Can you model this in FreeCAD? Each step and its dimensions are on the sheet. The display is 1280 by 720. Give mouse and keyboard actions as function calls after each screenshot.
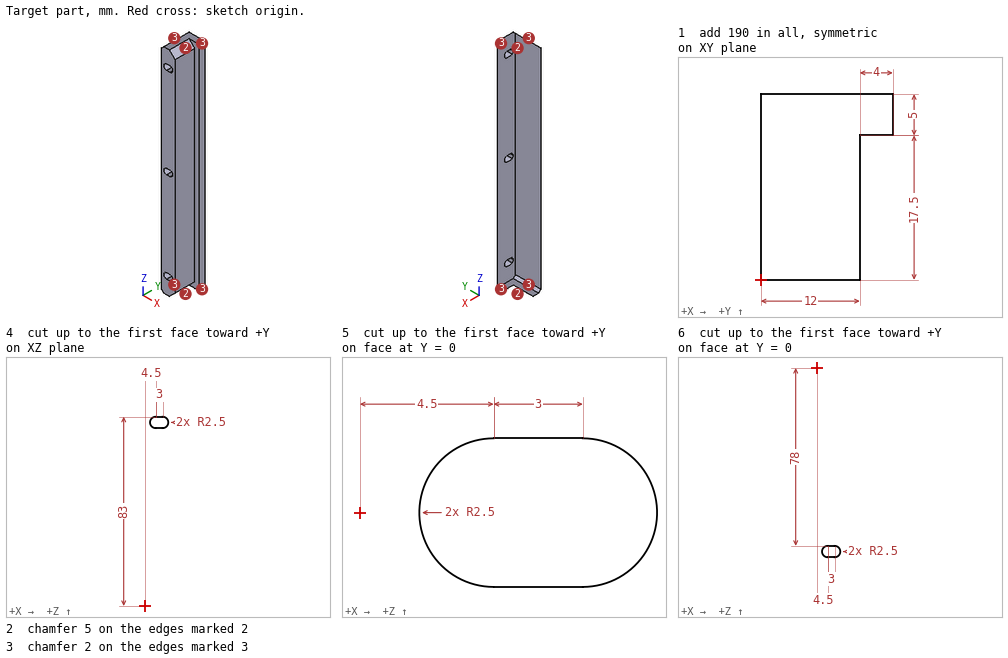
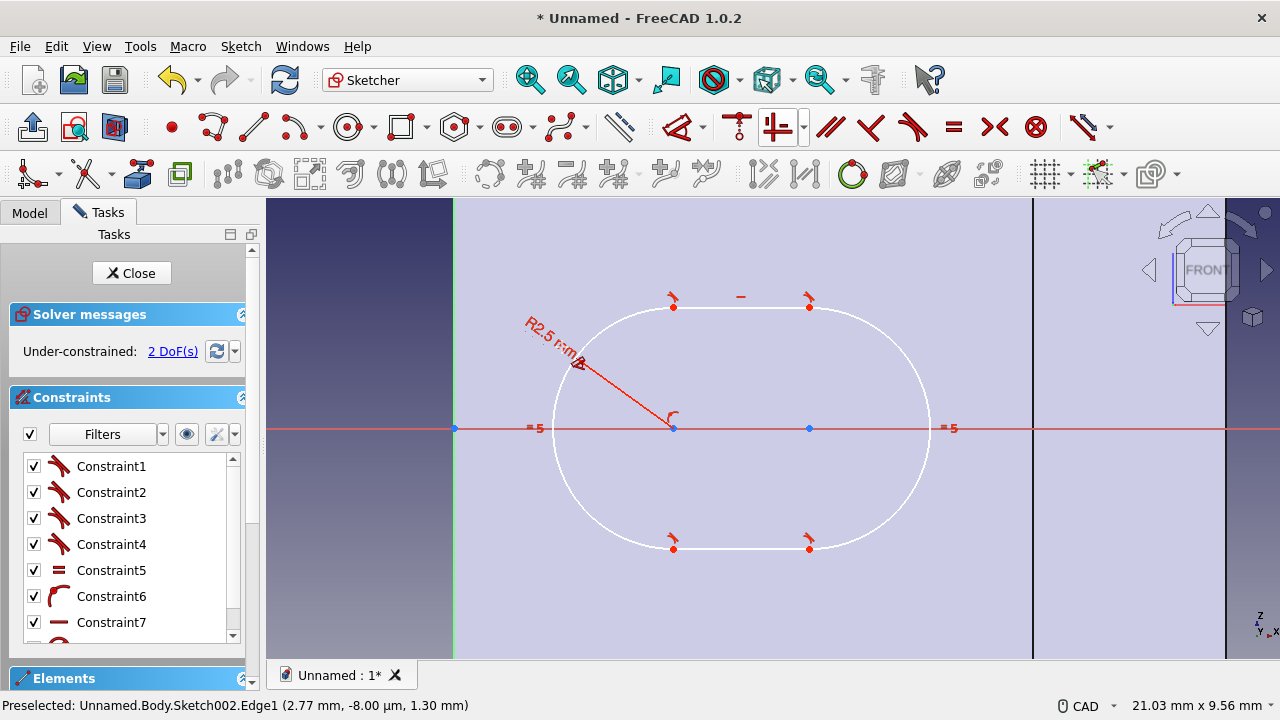
click(714, 308)
click(742, 274)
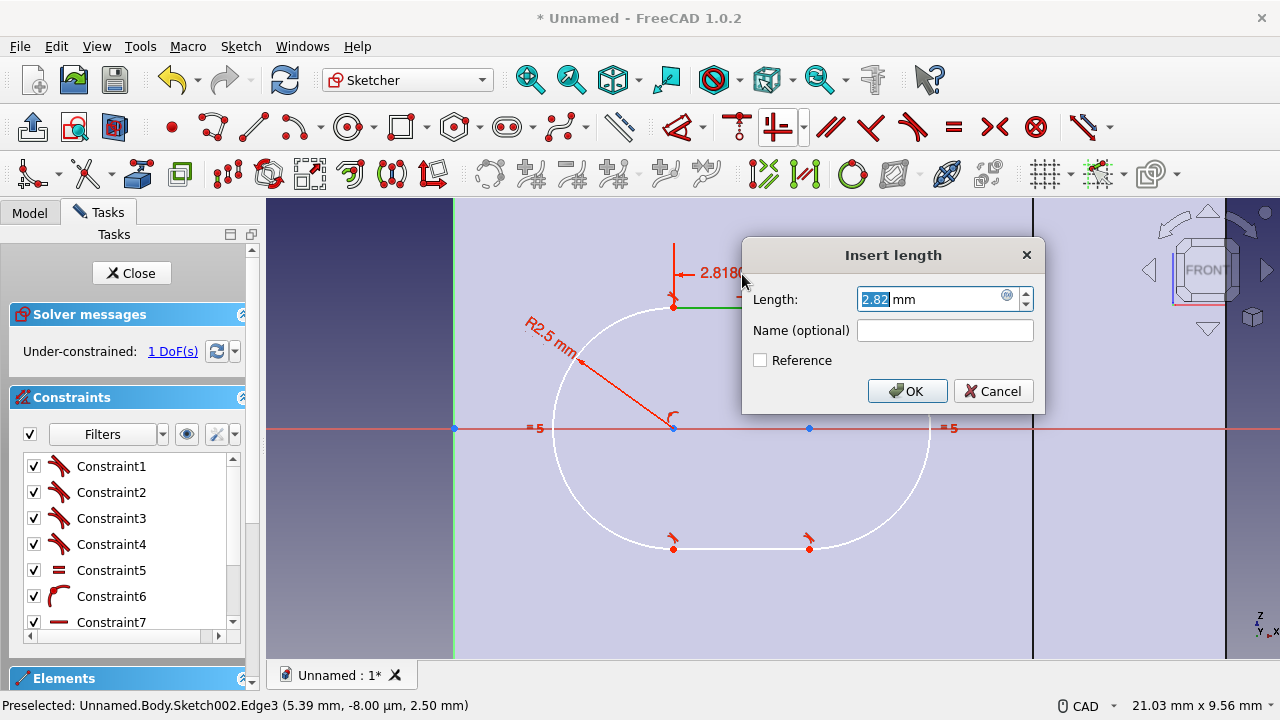
text(3)
key(Return)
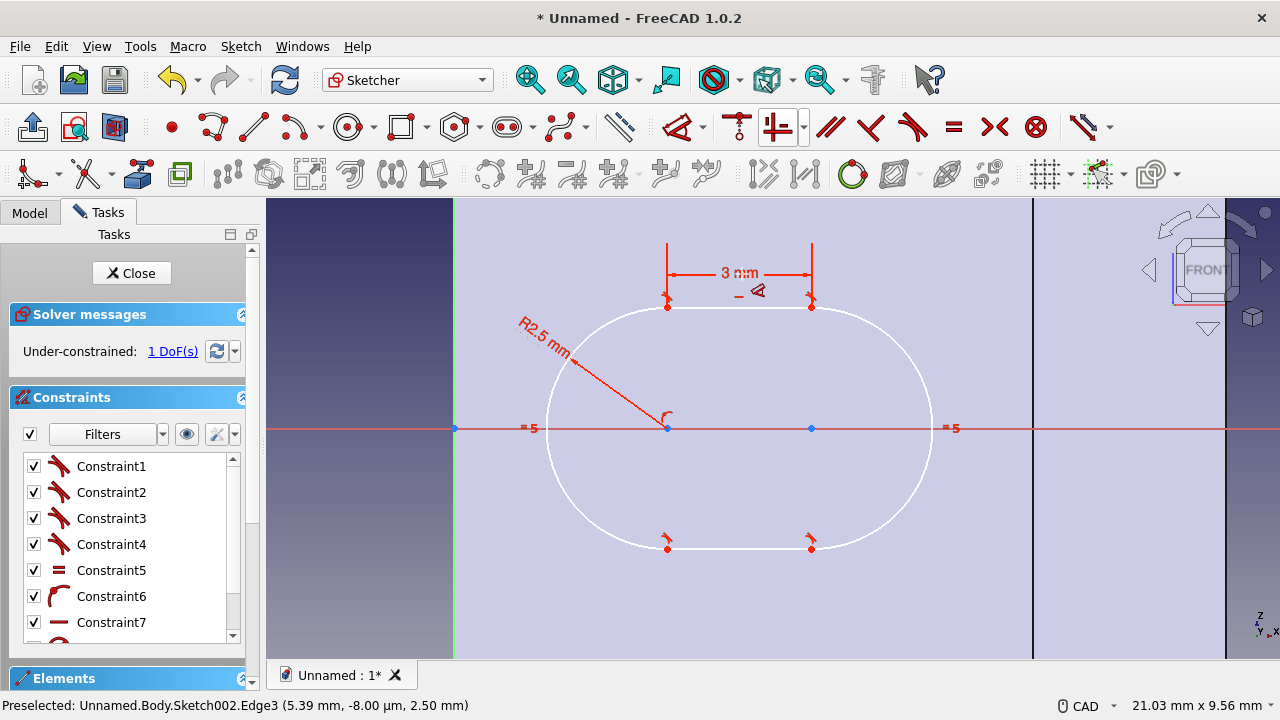
click(667, 308)
click(561, 274)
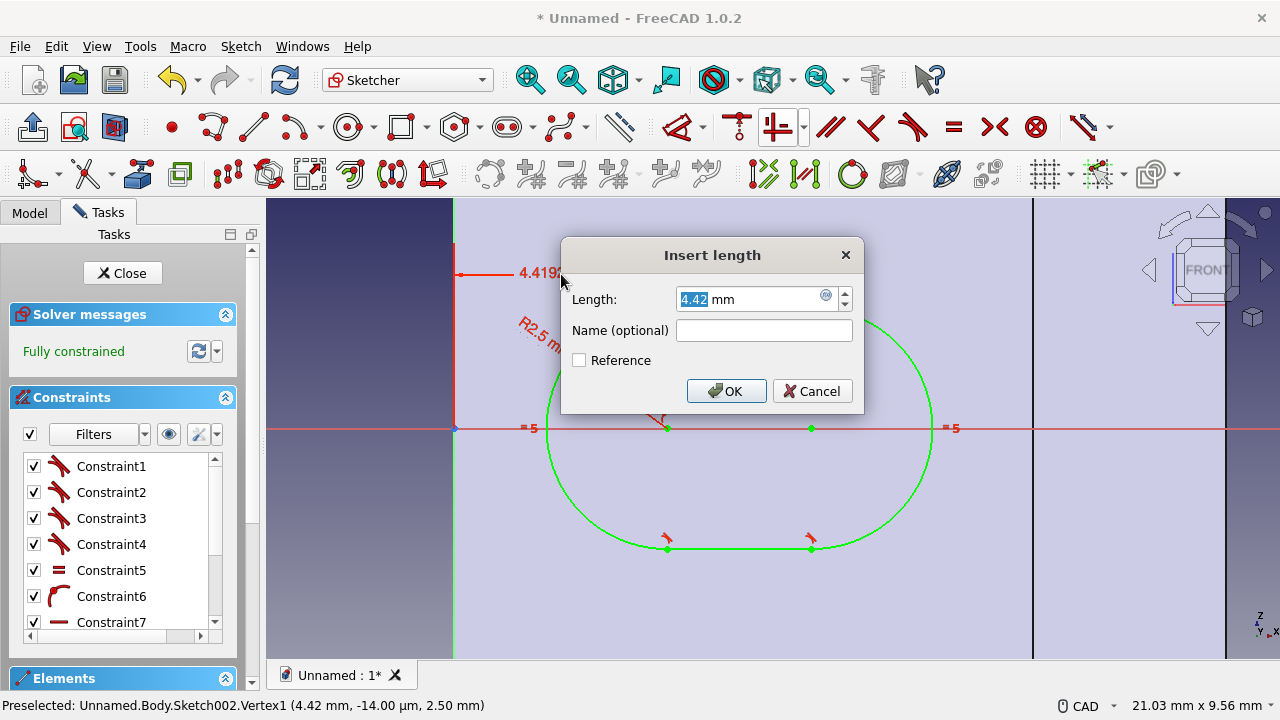
text(4.5)
key(Return)
key(Escape)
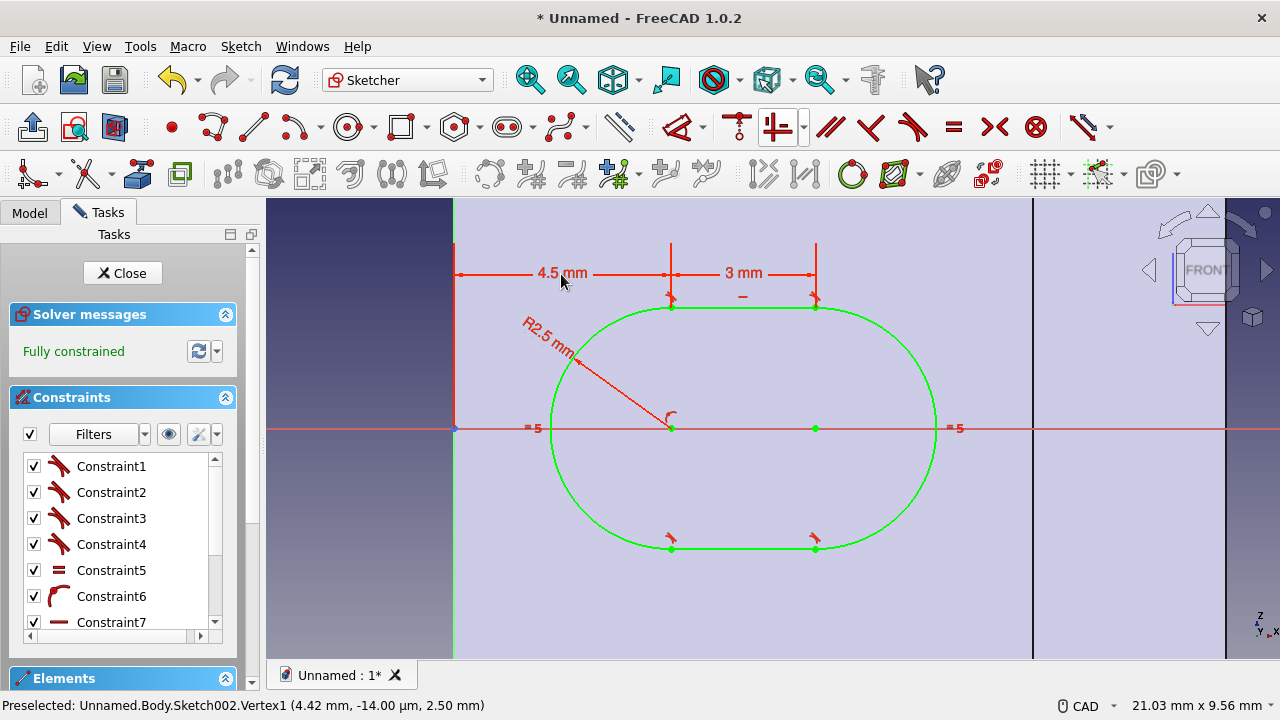
click(123, 273)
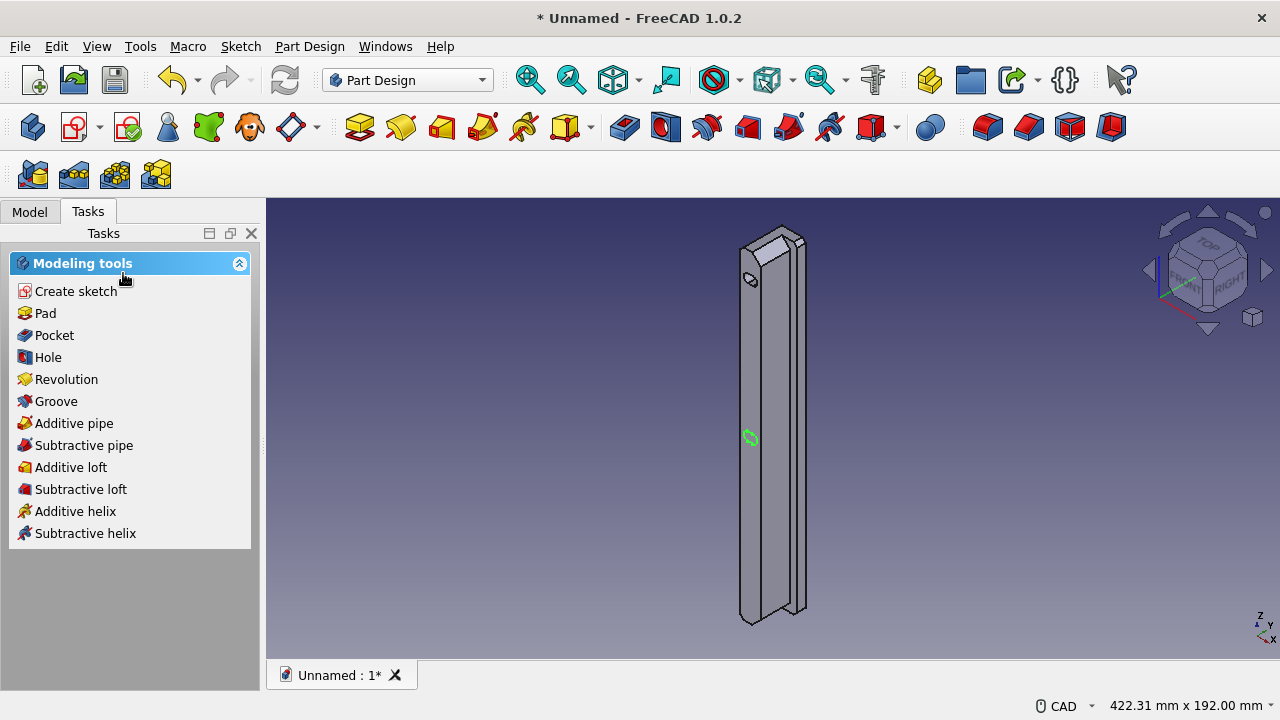
click(625, 128)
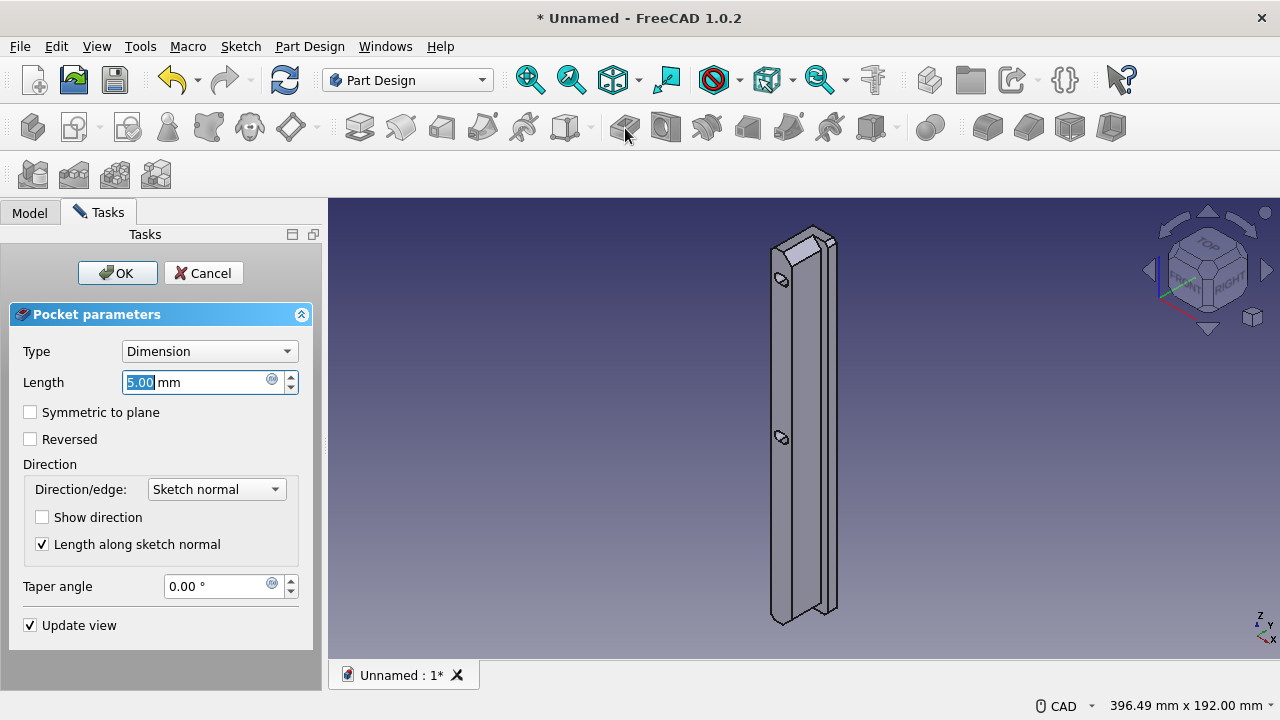
click(210, 352)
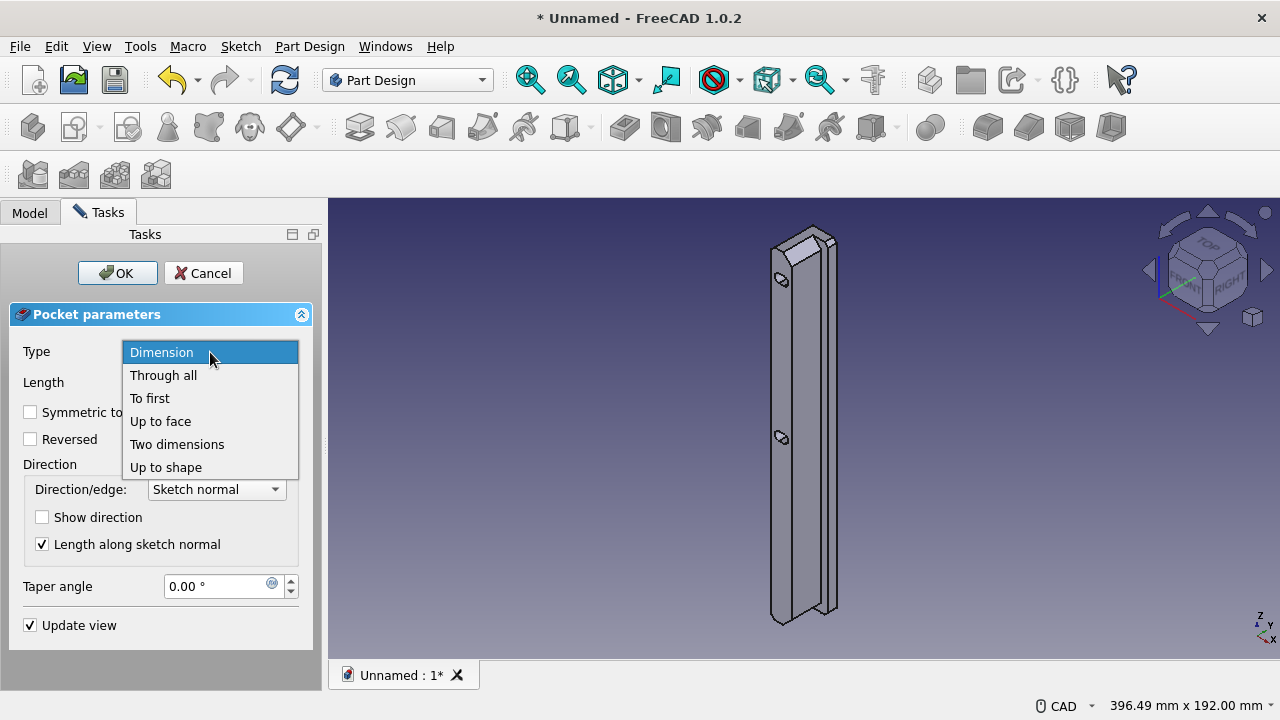
click(208, 398)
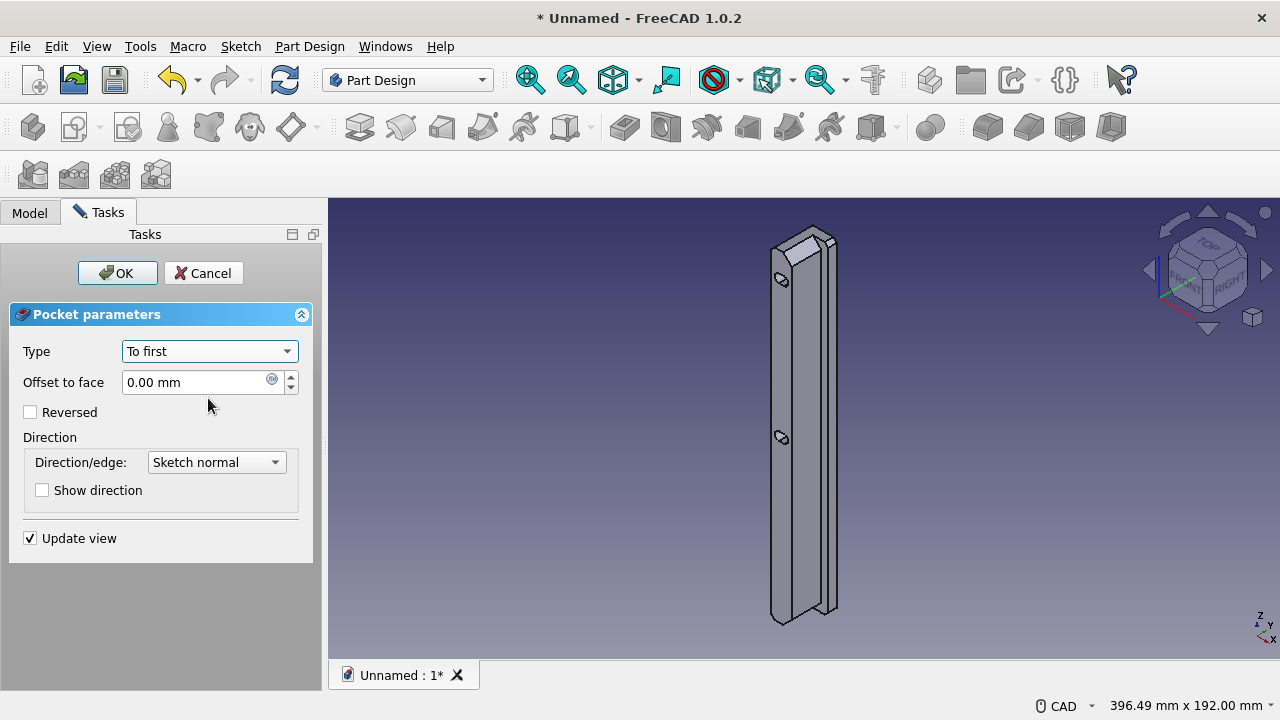
click(118, 273)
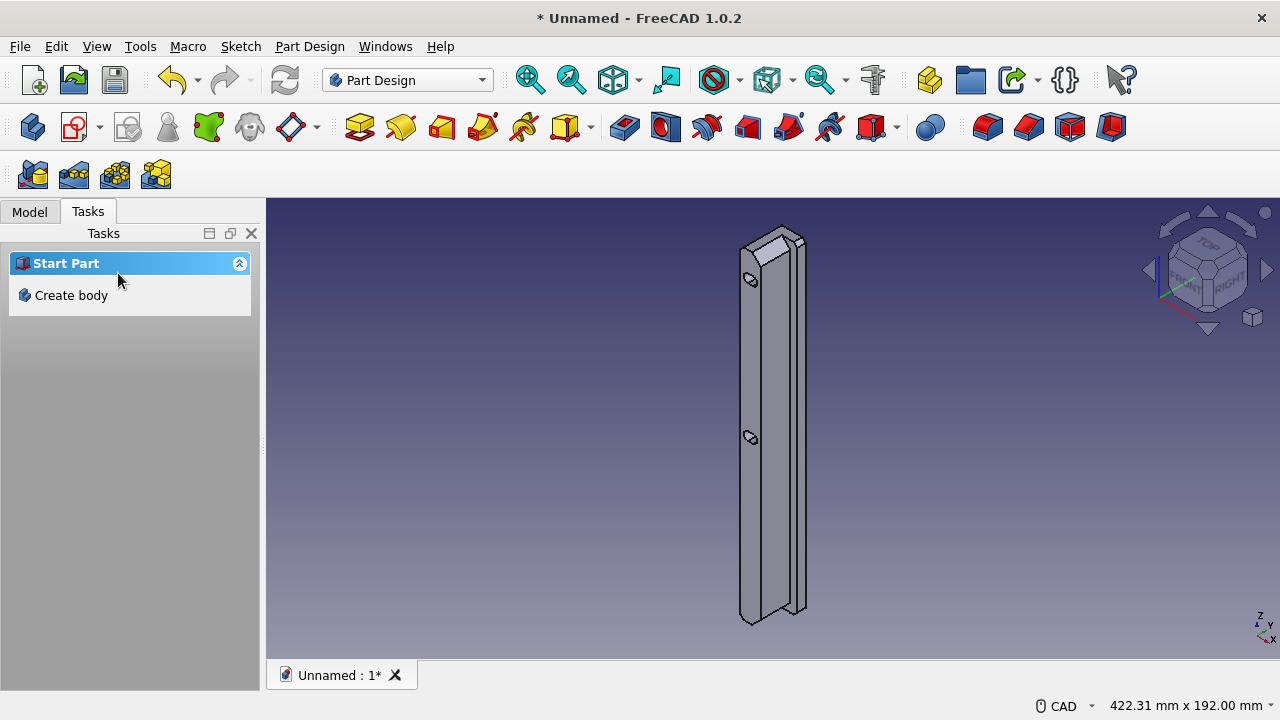
click(751, 330)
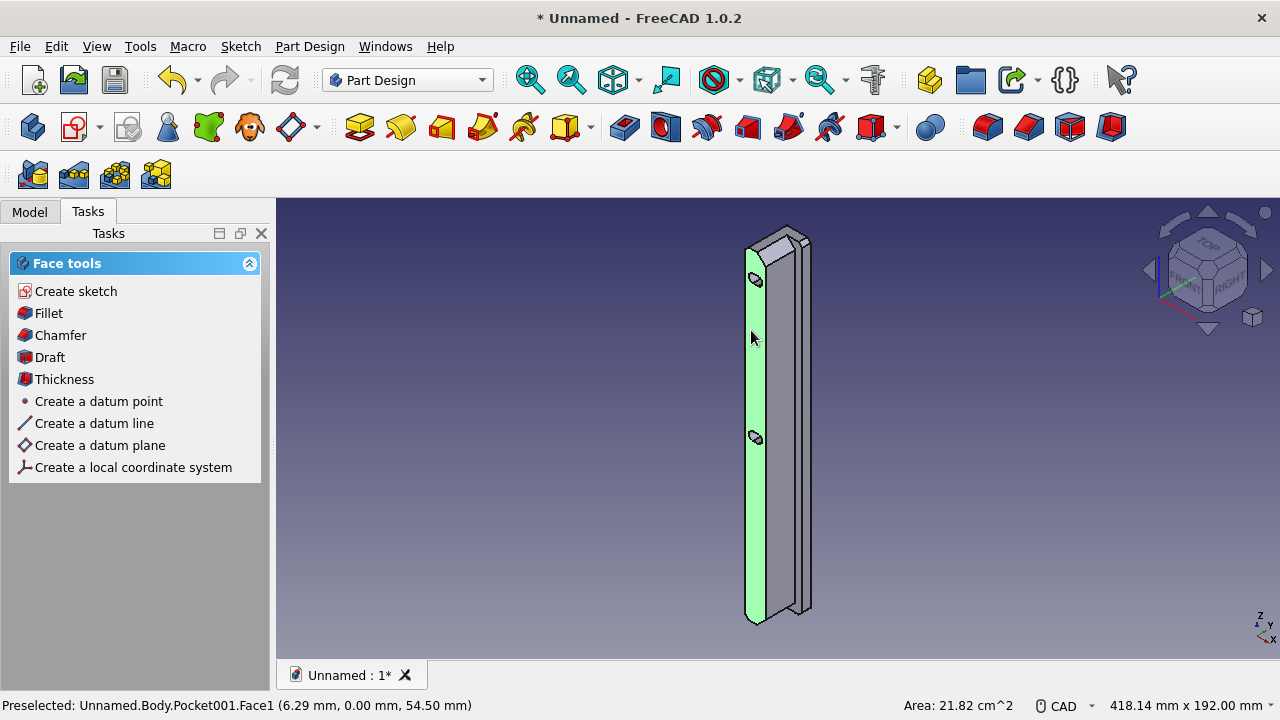
click(74, 128)